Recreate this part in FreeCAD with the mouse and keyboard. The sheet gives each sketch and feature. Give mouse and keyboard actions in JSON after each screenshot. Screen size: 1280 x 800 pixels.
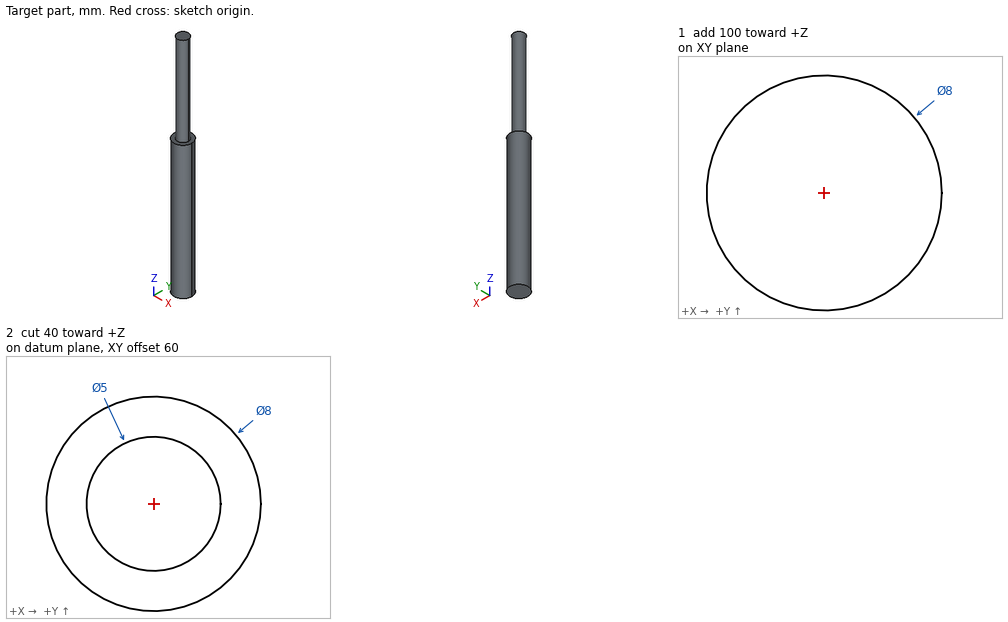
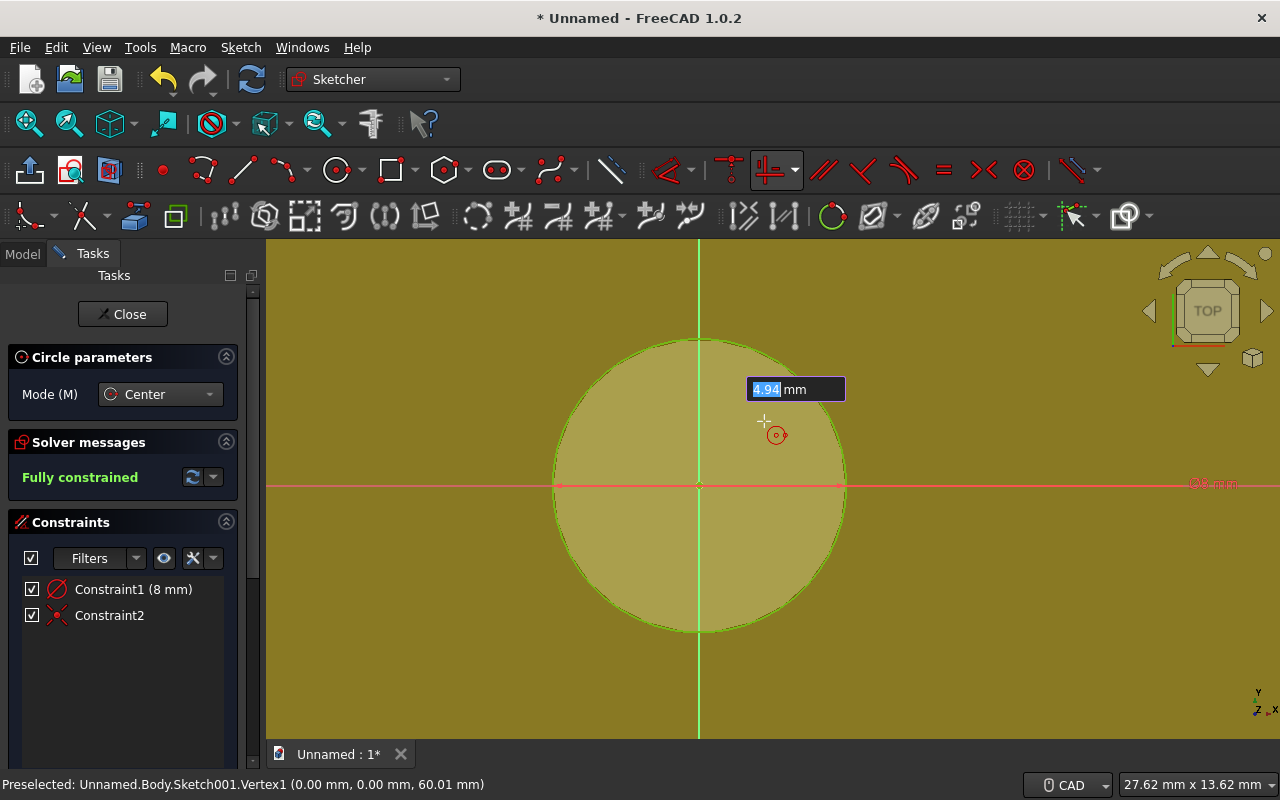
{"action": "type", "text": "5"}
{"action": "key", "text": "Return"}
{"action": "key", "text": "Escape"}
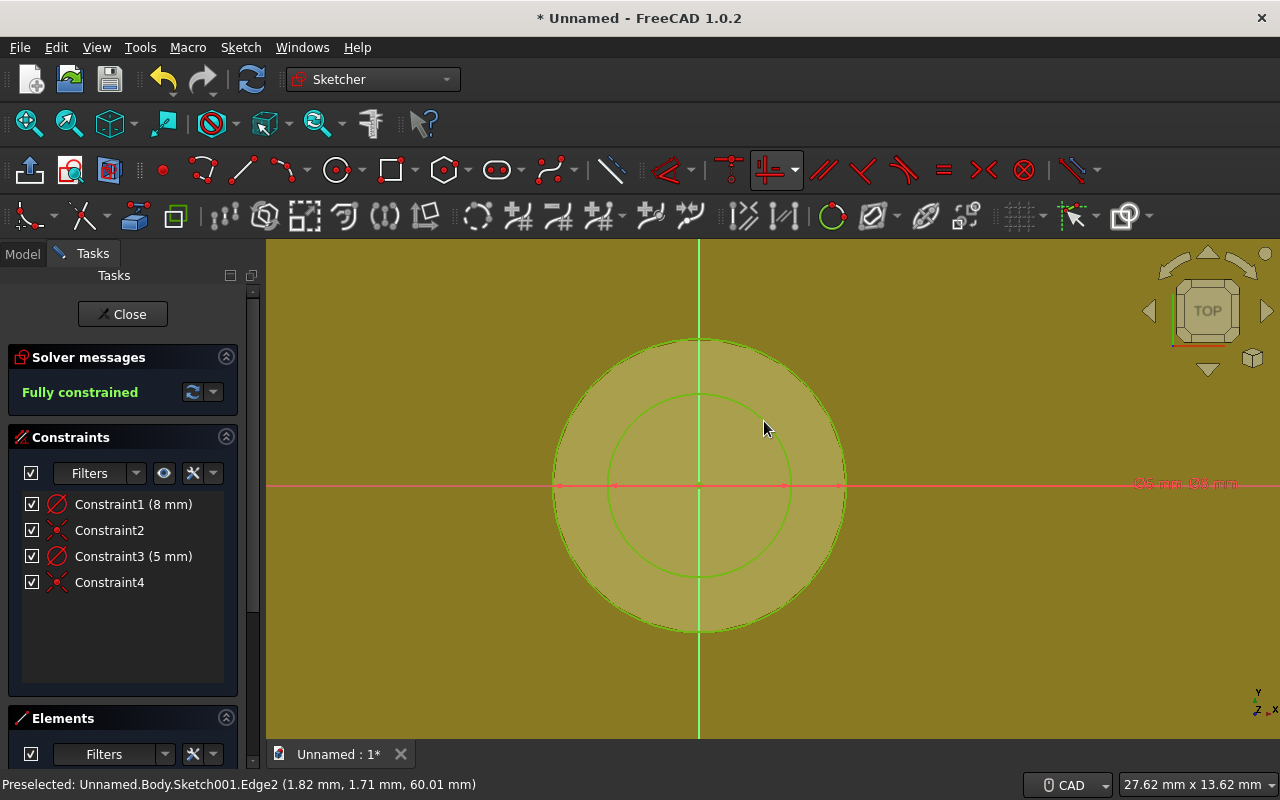
{"action": "left_click", "coordinate": [123, 314]}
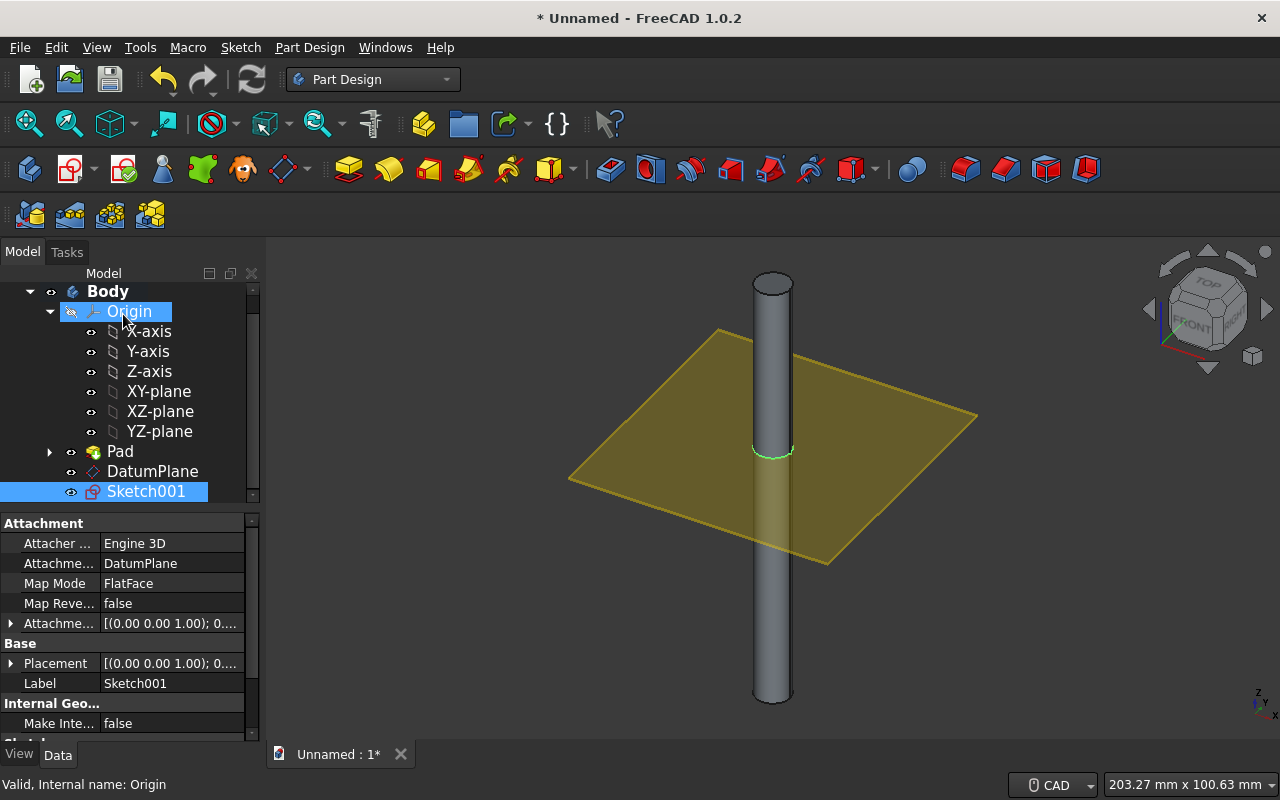
{"action": "left_click", "coordinate": [612, 170]}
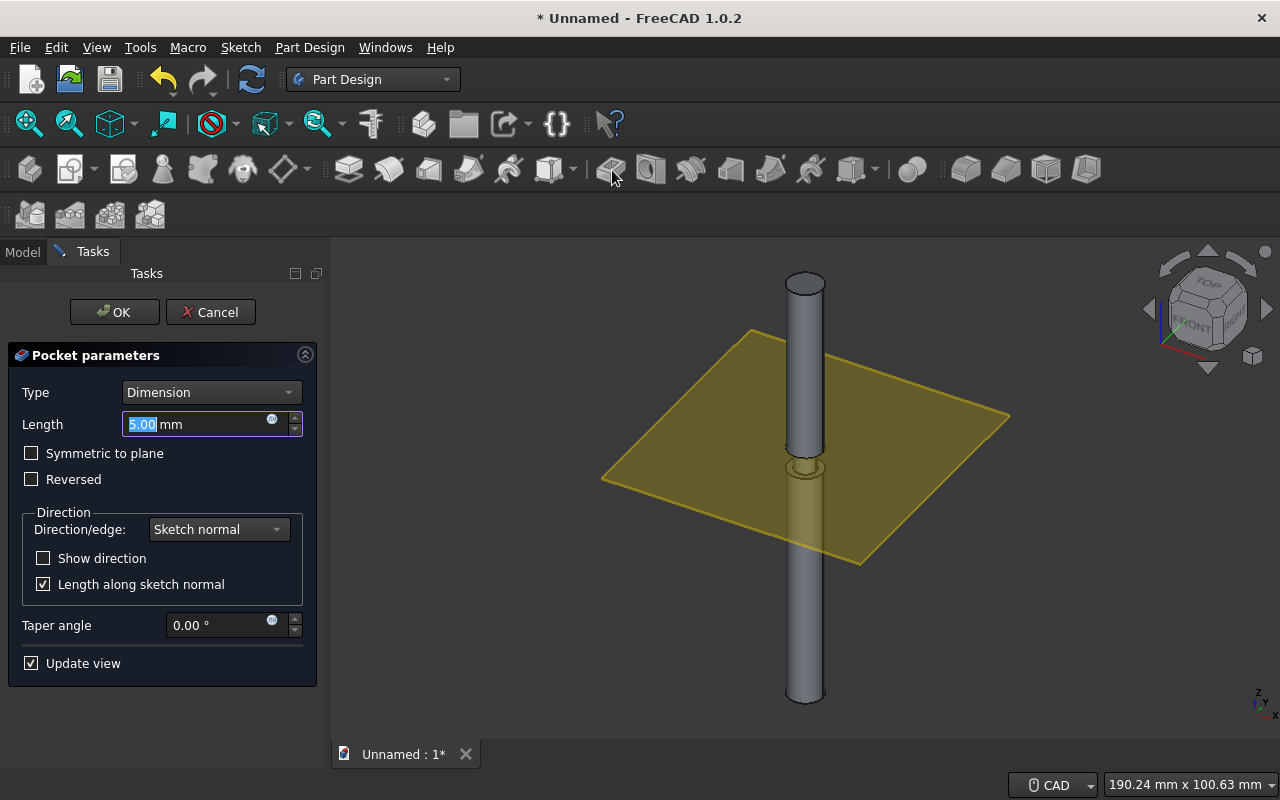
{"action": "type", "text": "40"}
{"action": "key", "text": "Tab"}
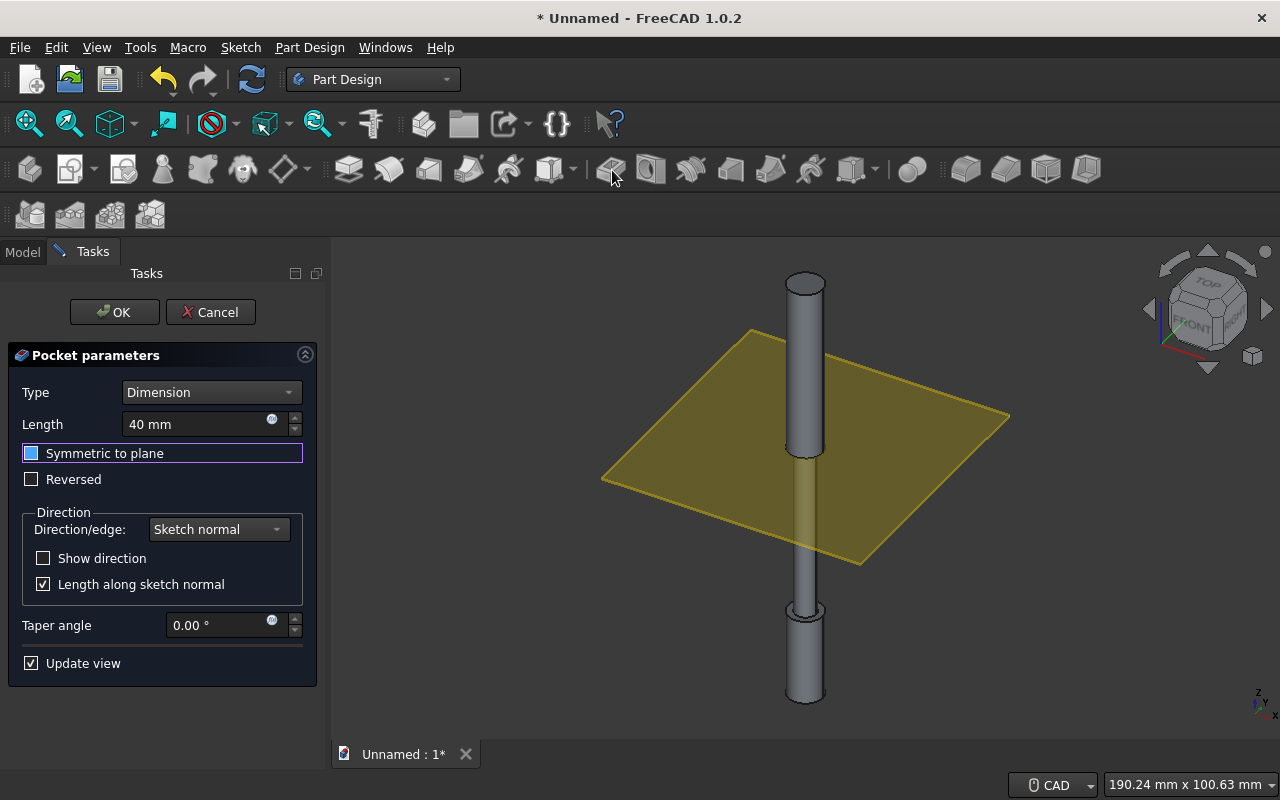
{"action": "left_click", "coordinate": [30, 479]}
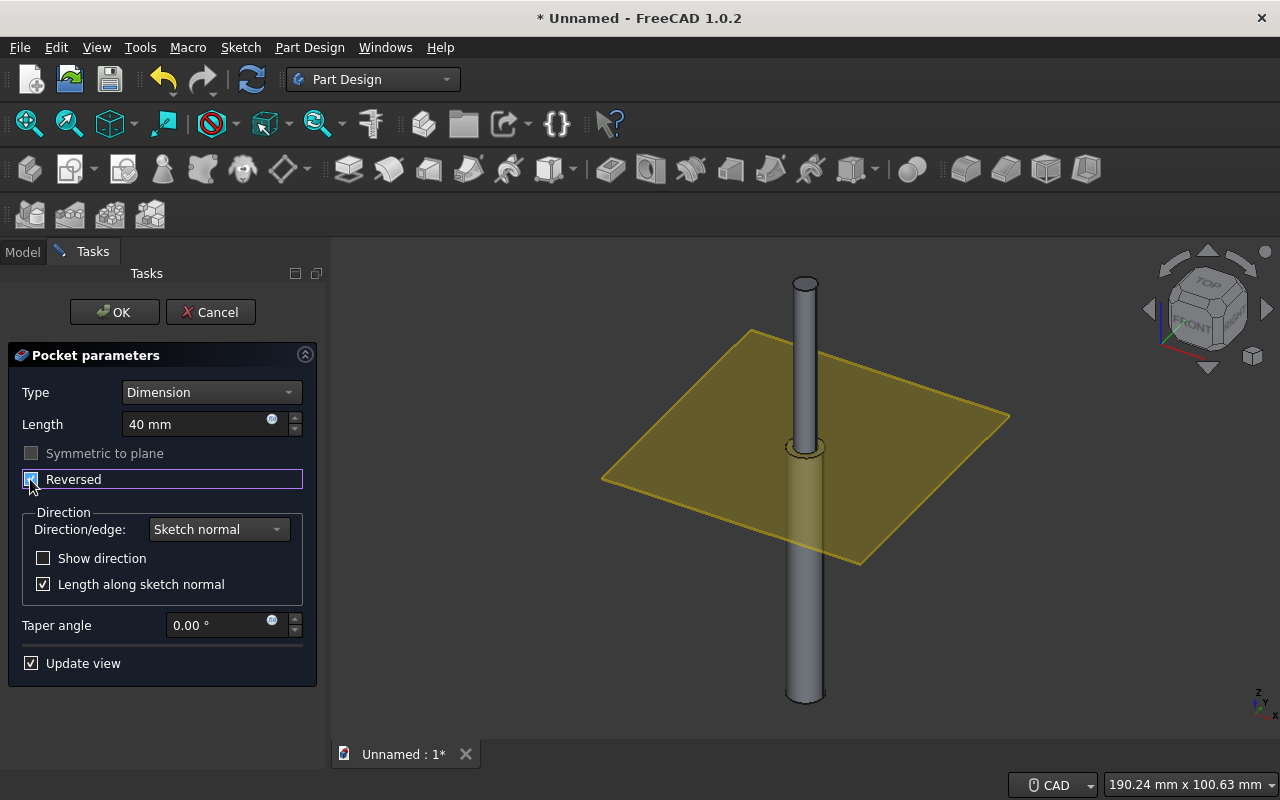
{"action": "left_click", "coordinate": [115, 312]}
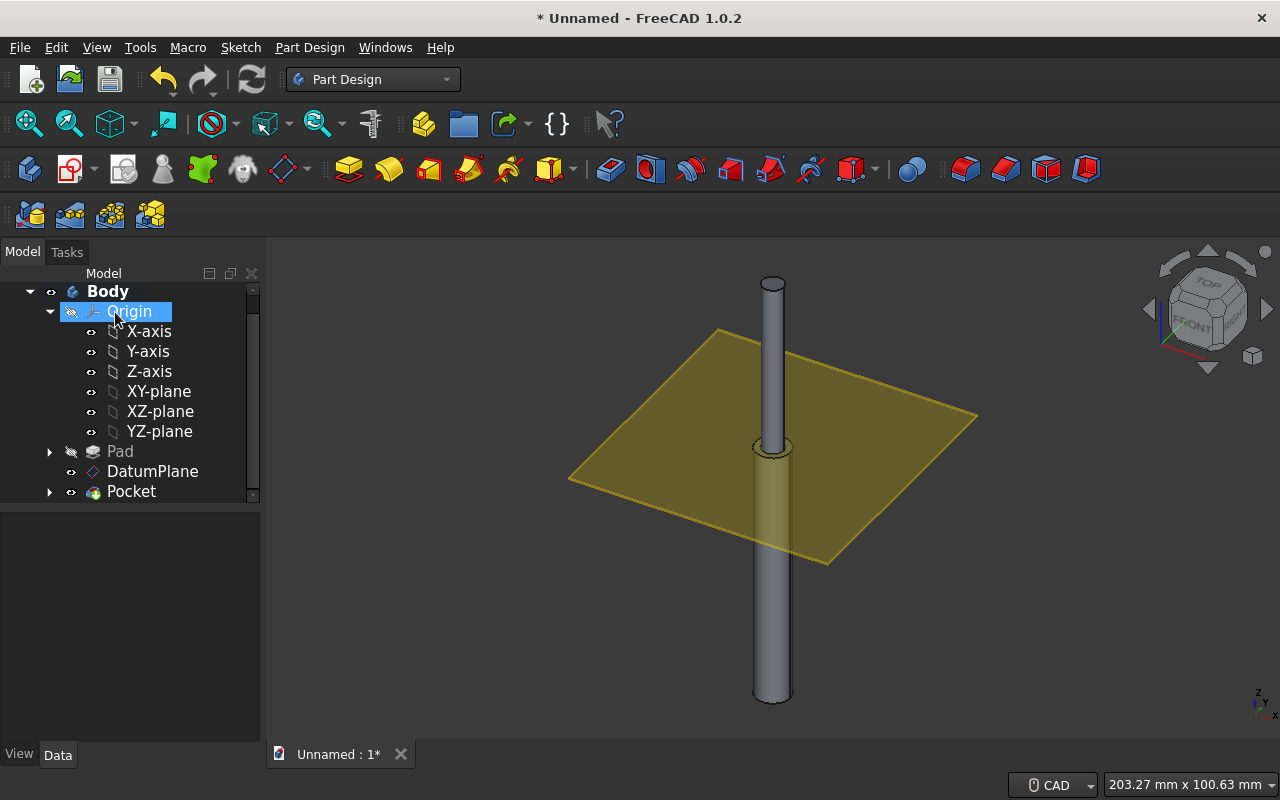
{"action": "left_click", "coordinate": [116, 472]}
{"action": "key", "text": "space"}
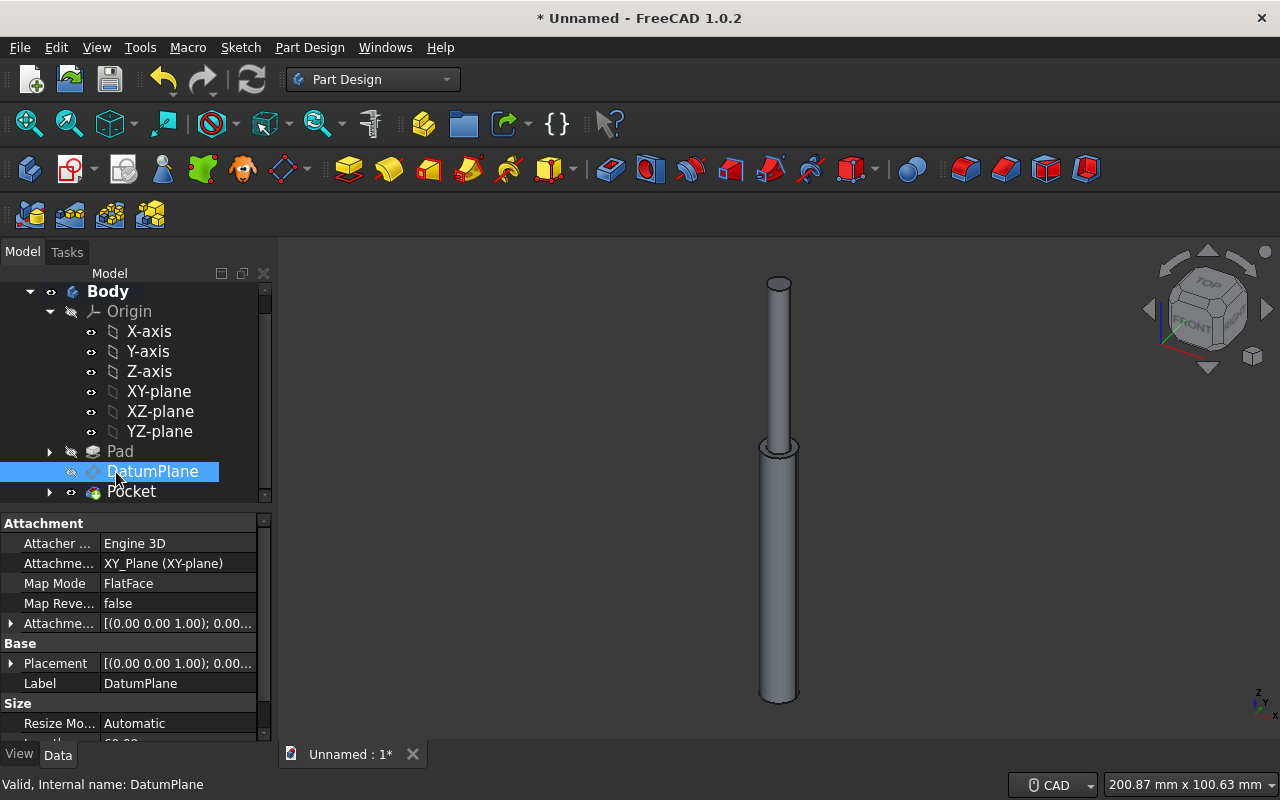
{"action": "key", "text": "0"}